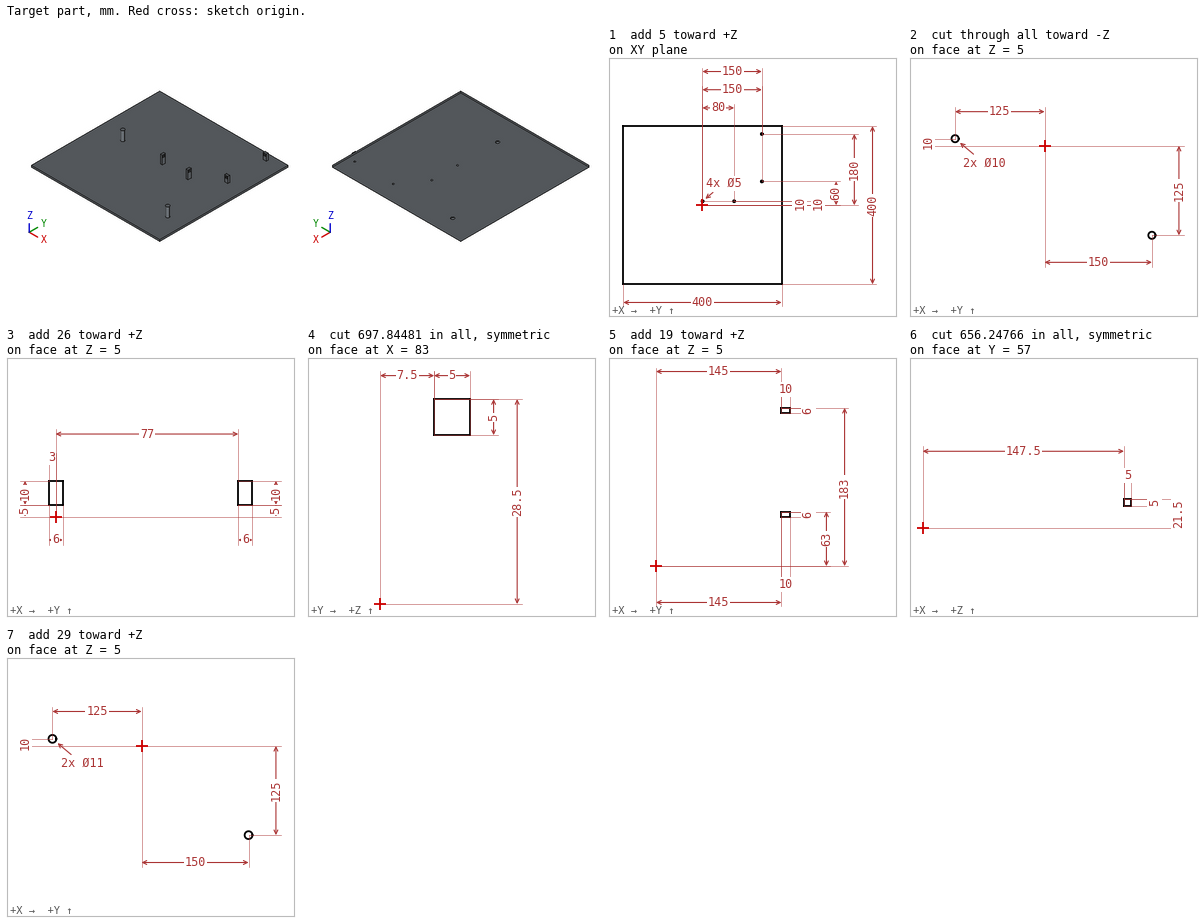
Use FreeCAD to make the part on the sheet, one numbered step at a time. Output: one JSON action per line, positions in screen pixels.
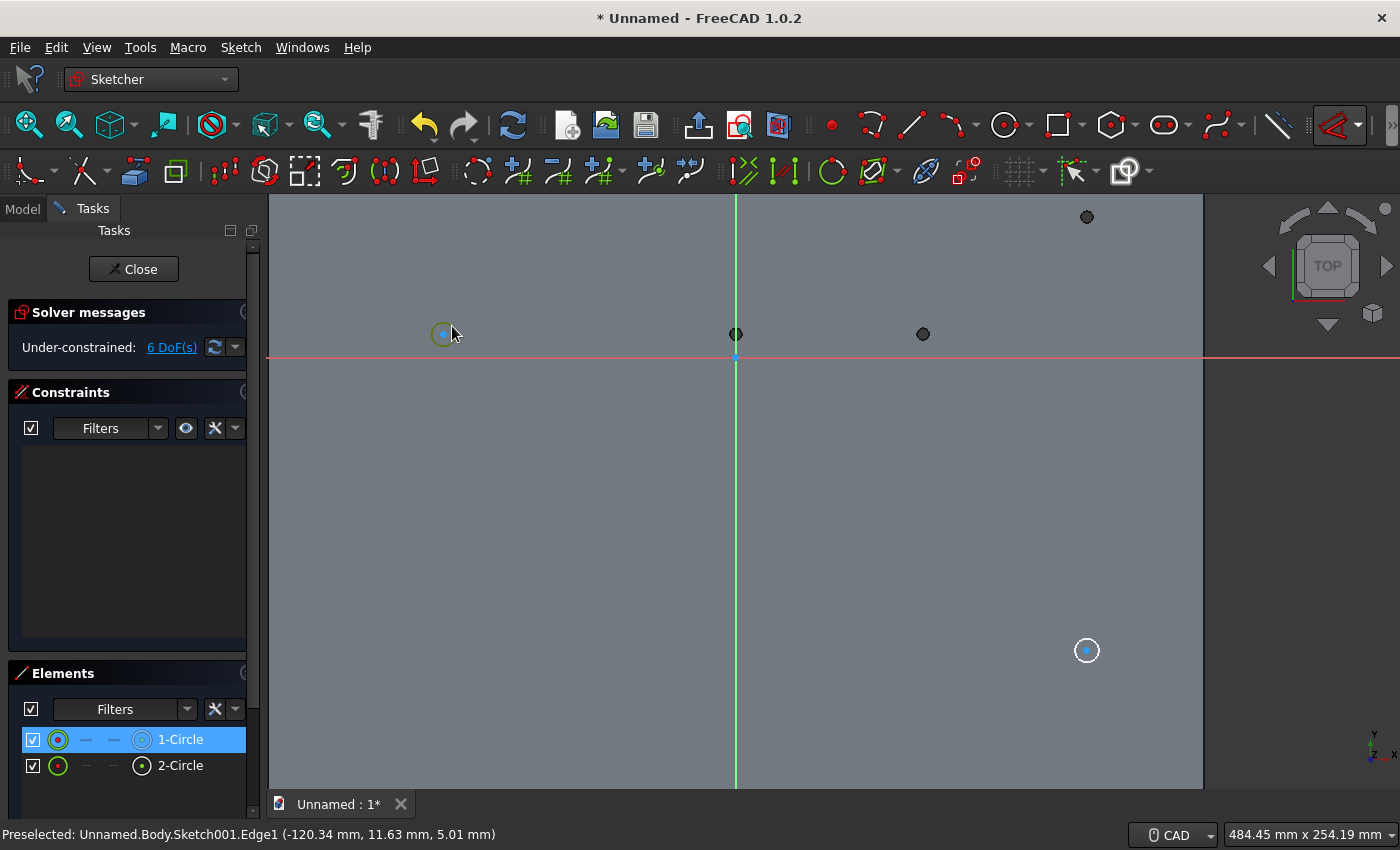
{"action": "left_click", "coordinate": [1095, 642]}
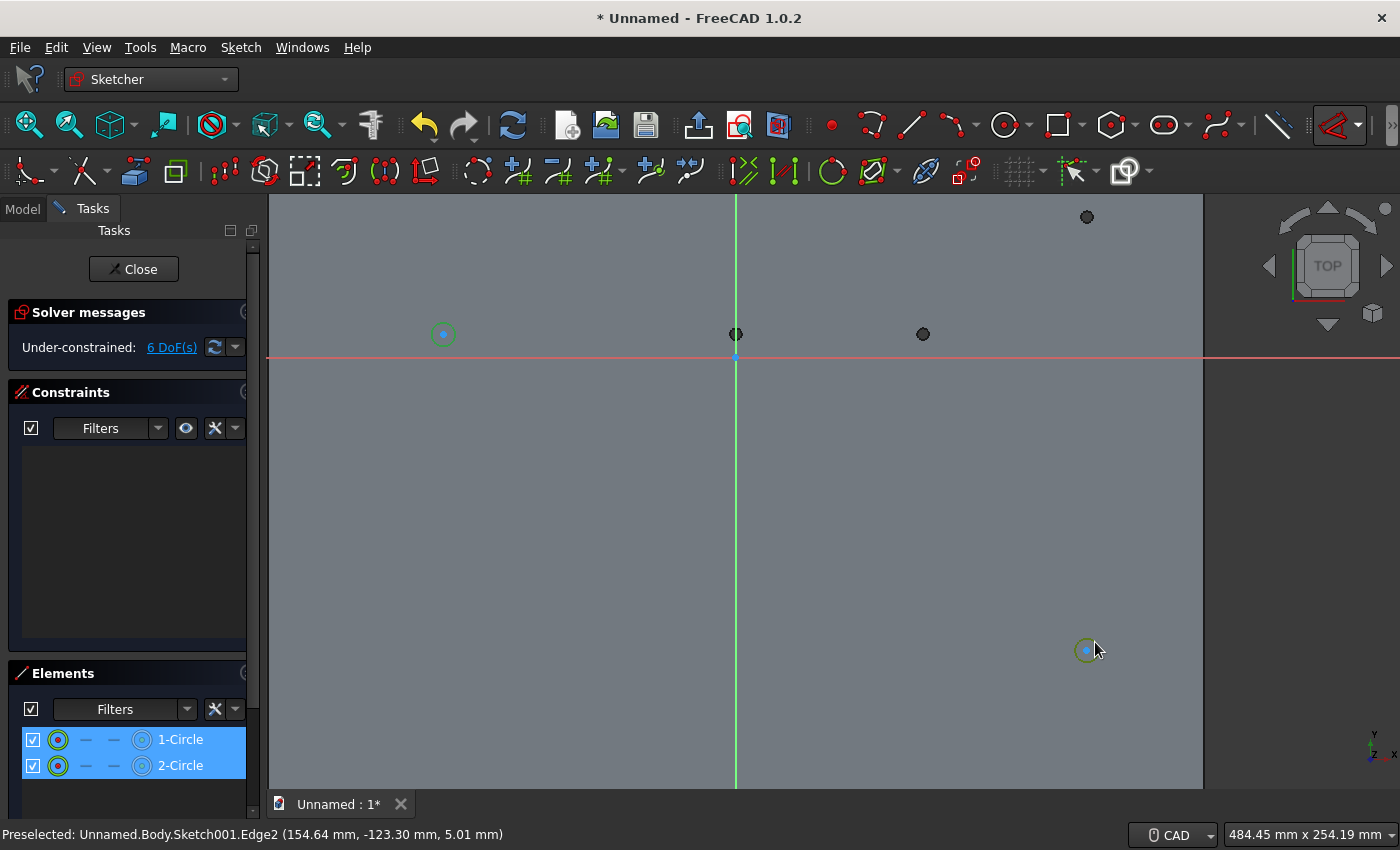
{"action": "key", "text": "e"}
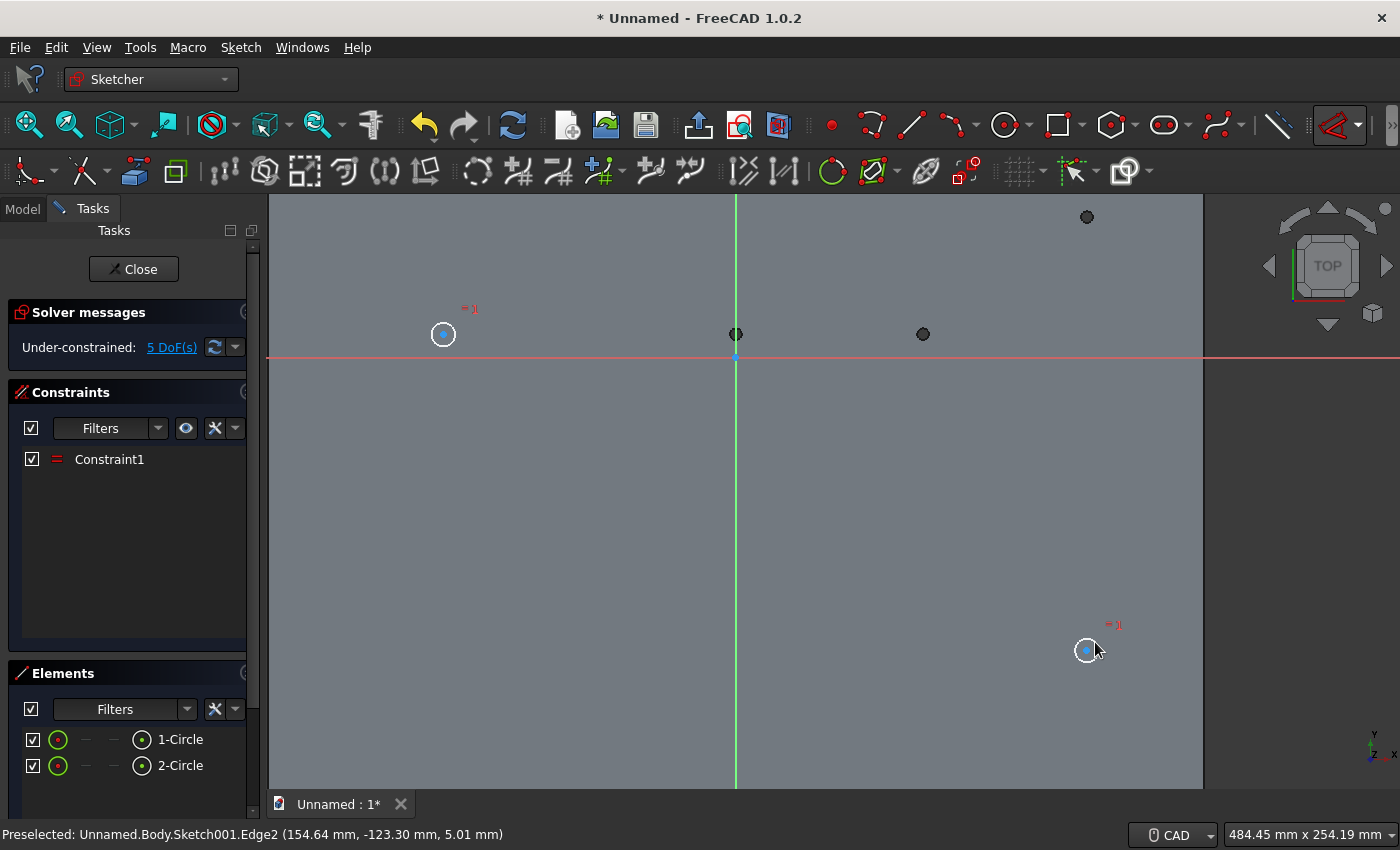
{"action": "scroll", "coordinate": [452, 326], "scroll_direction": "up", "scroll_amount": 3}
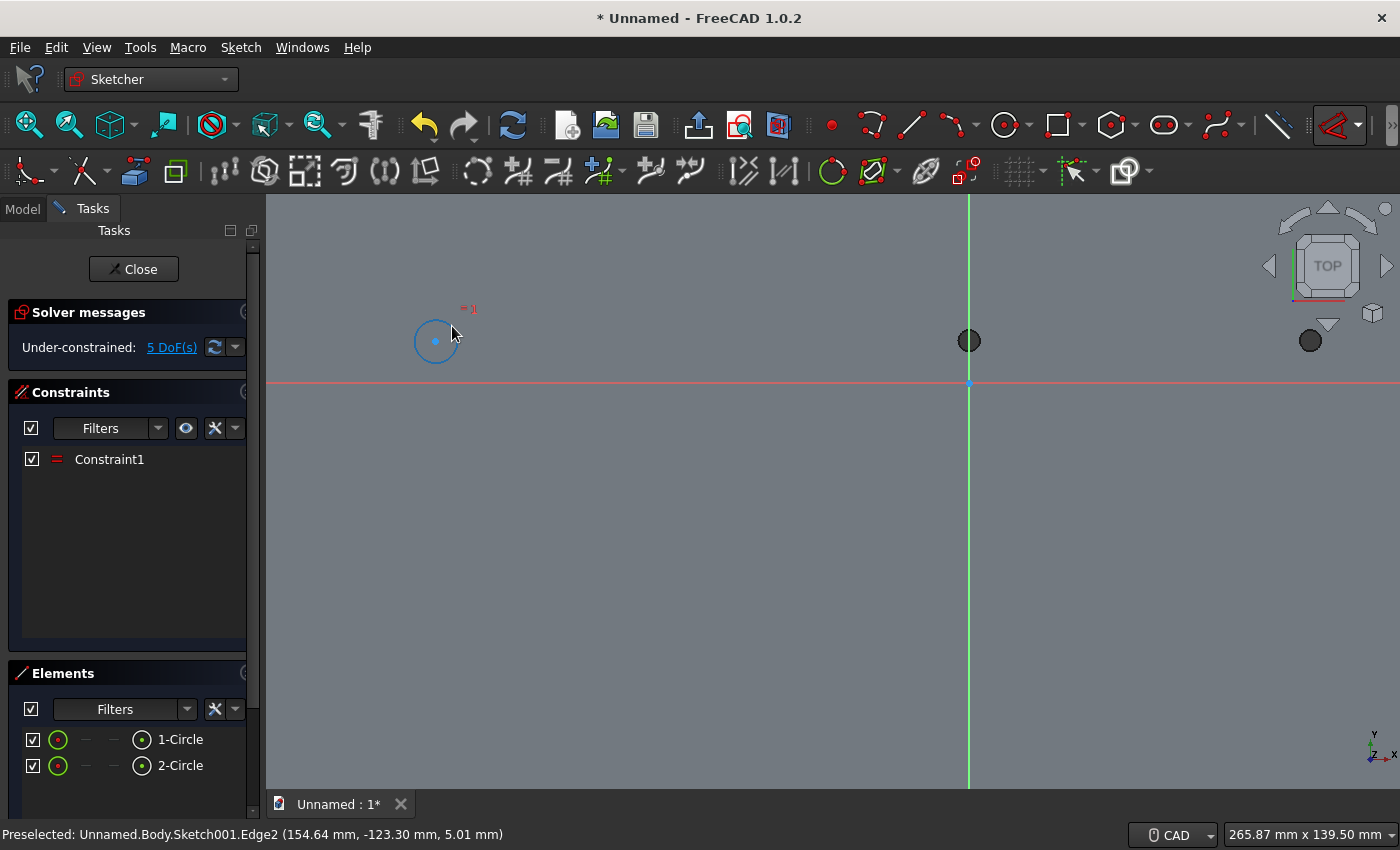
{"action": "left_click", "coordinate": [451, 326]}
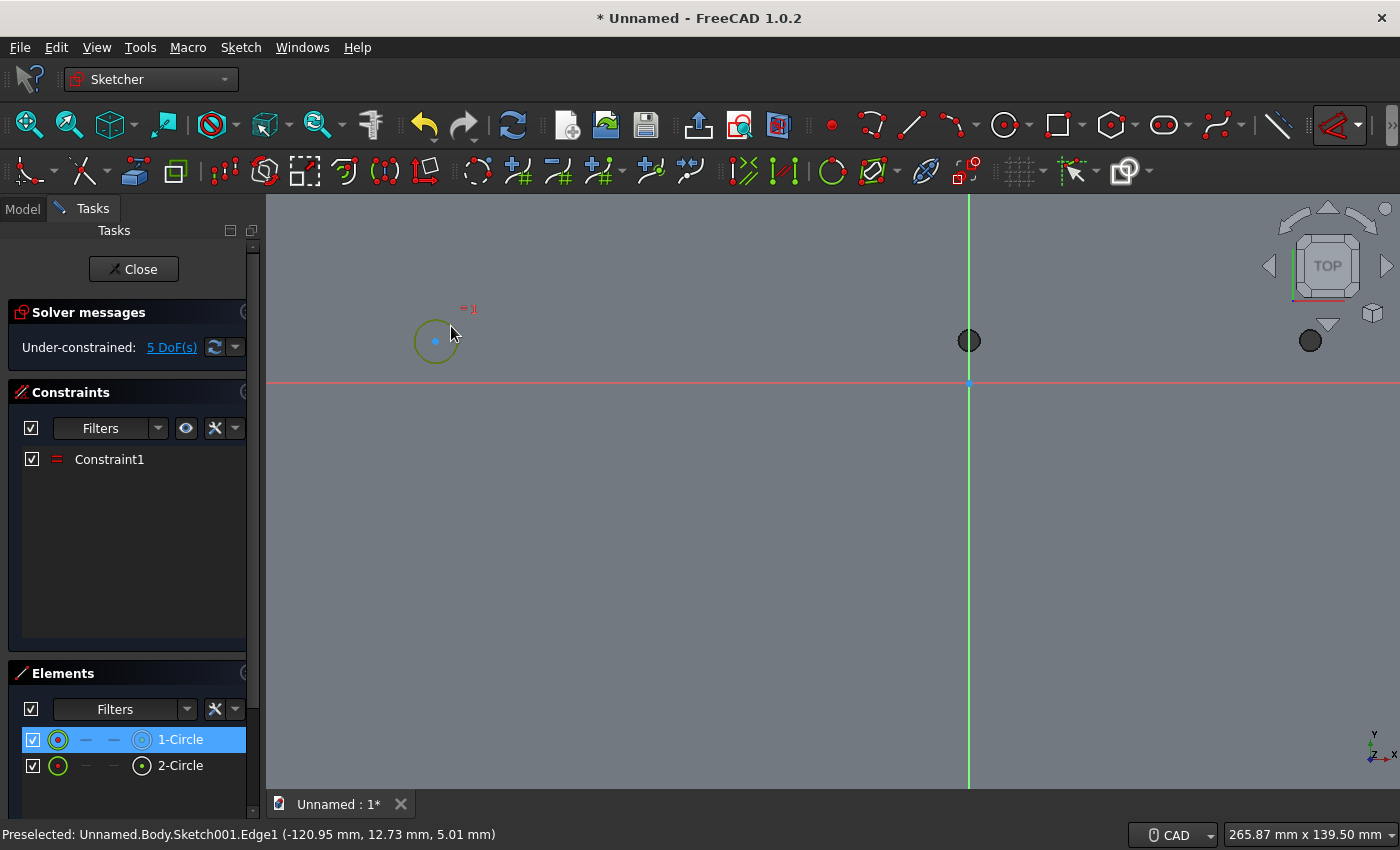
{"action": "key", "text": "k o"}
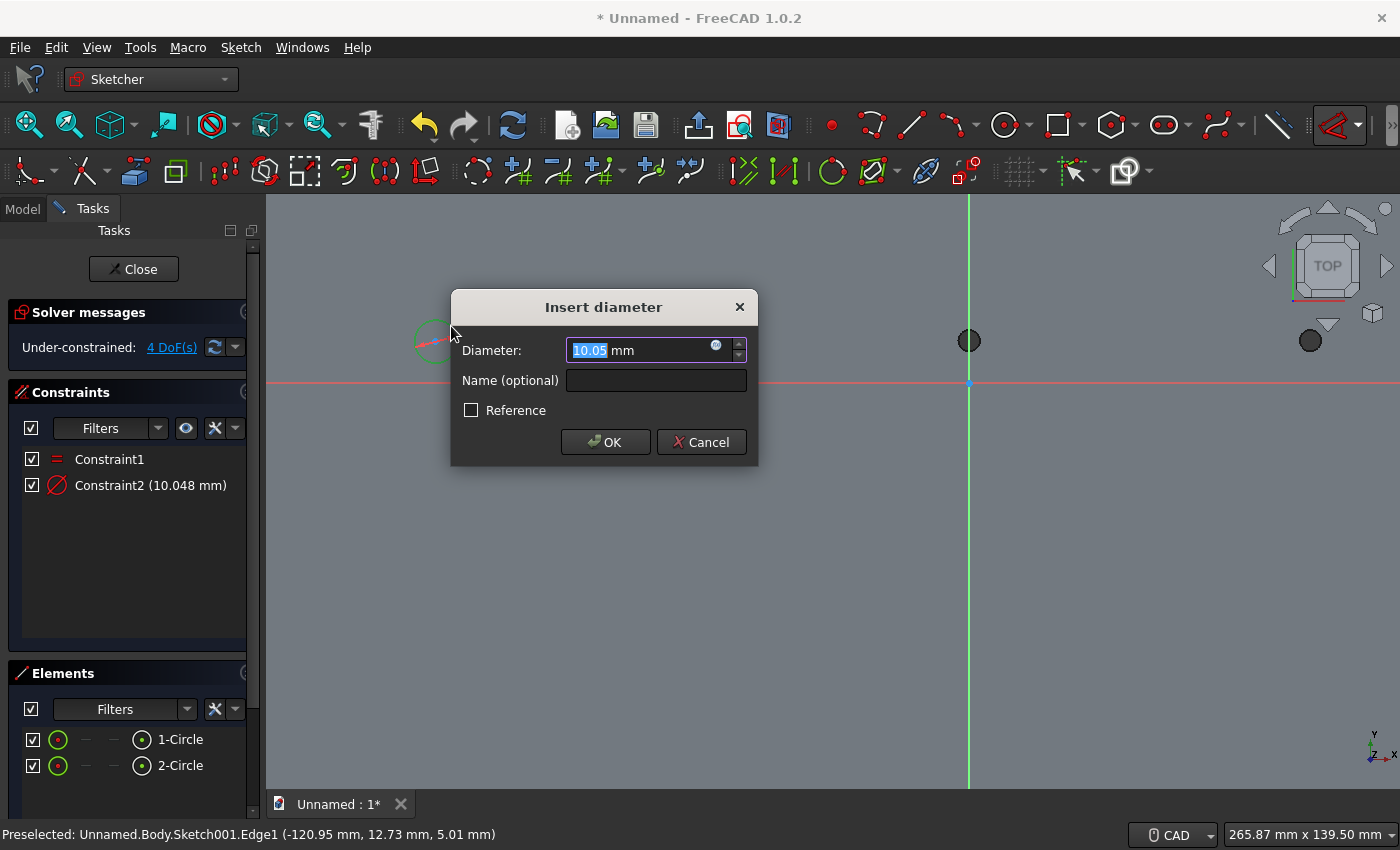
{"action": "type", "text": "10"}
{"action": "key", "text": "Return"}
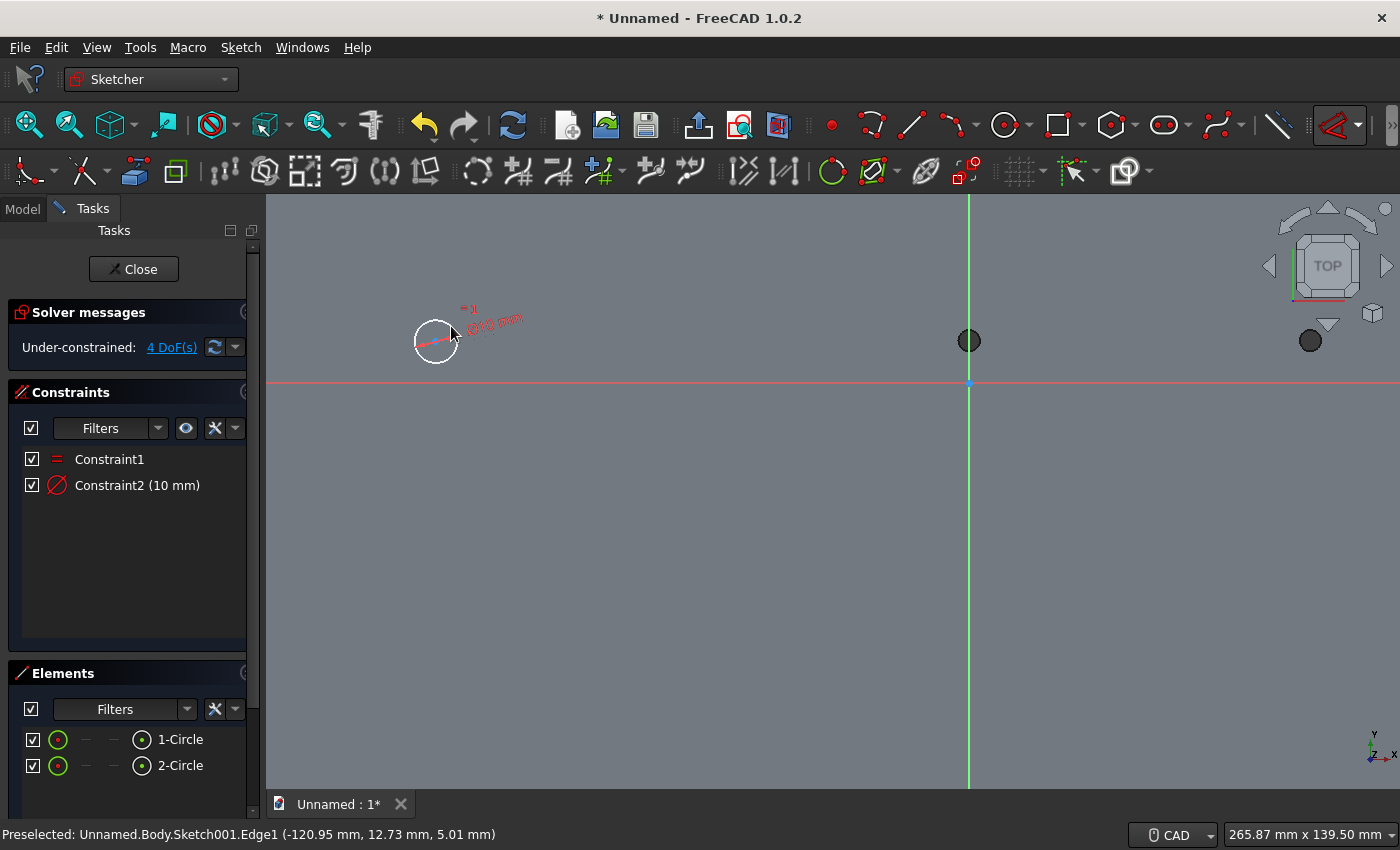
{"action": "left_click", "coordinate": [436, 342]}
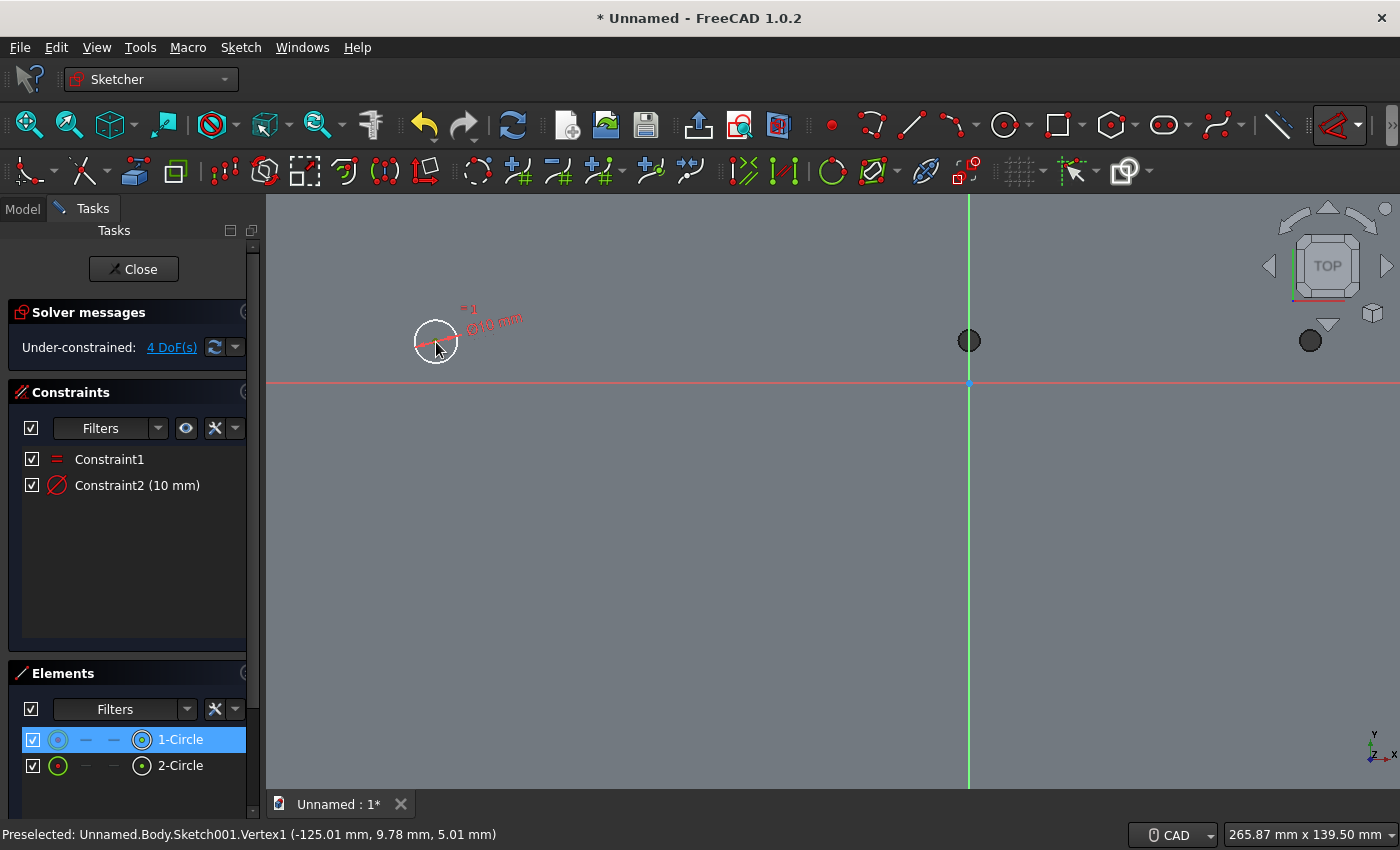
{"action": "key", "text": "i"}